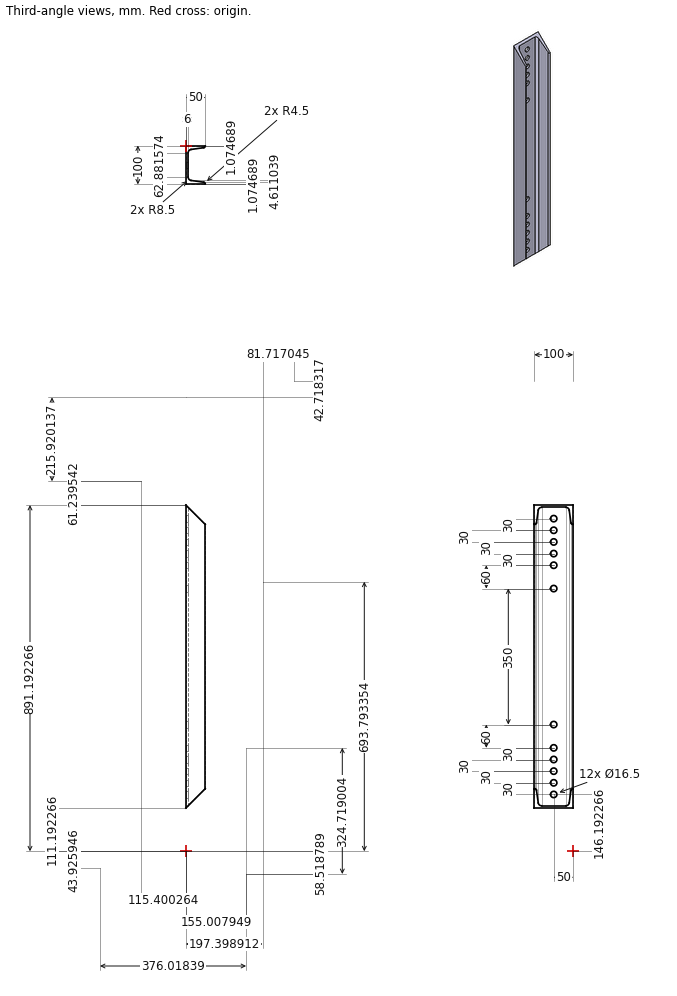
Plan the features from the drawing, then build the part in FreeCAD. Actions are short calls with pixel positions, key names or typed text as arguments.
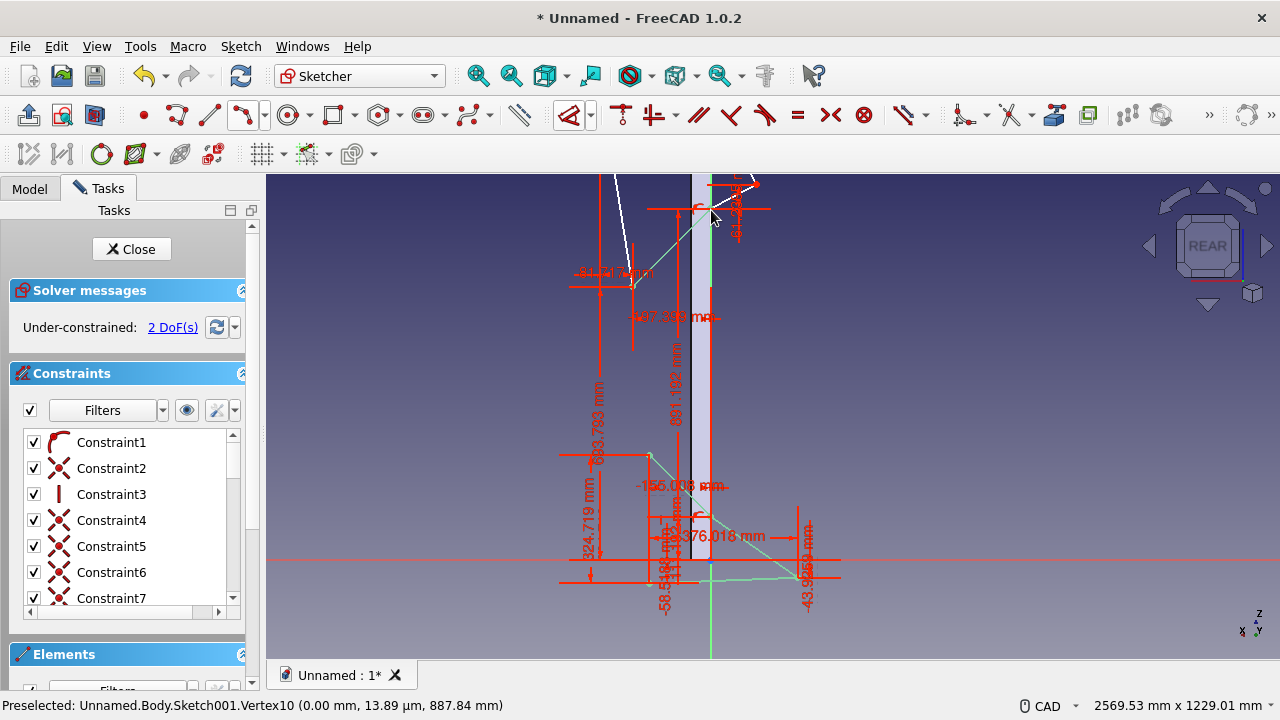
scroll(711, 518, down, 3)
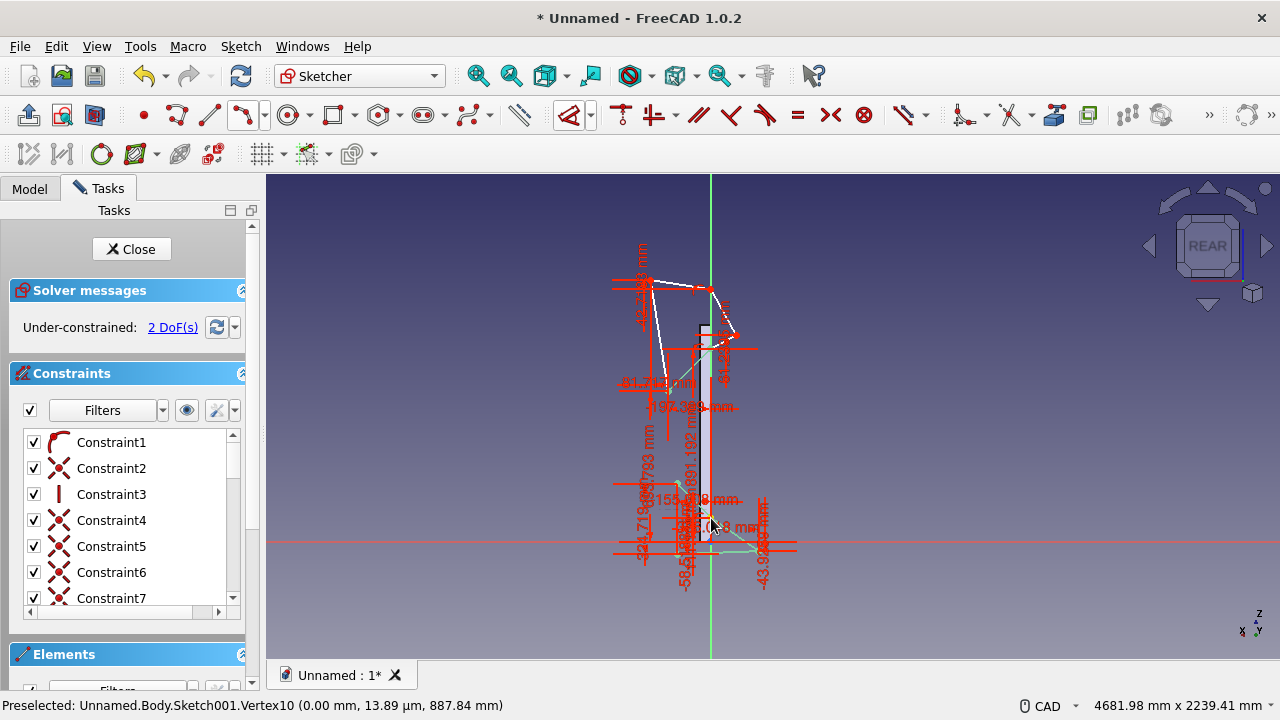
scroll(736, 335, up, 3)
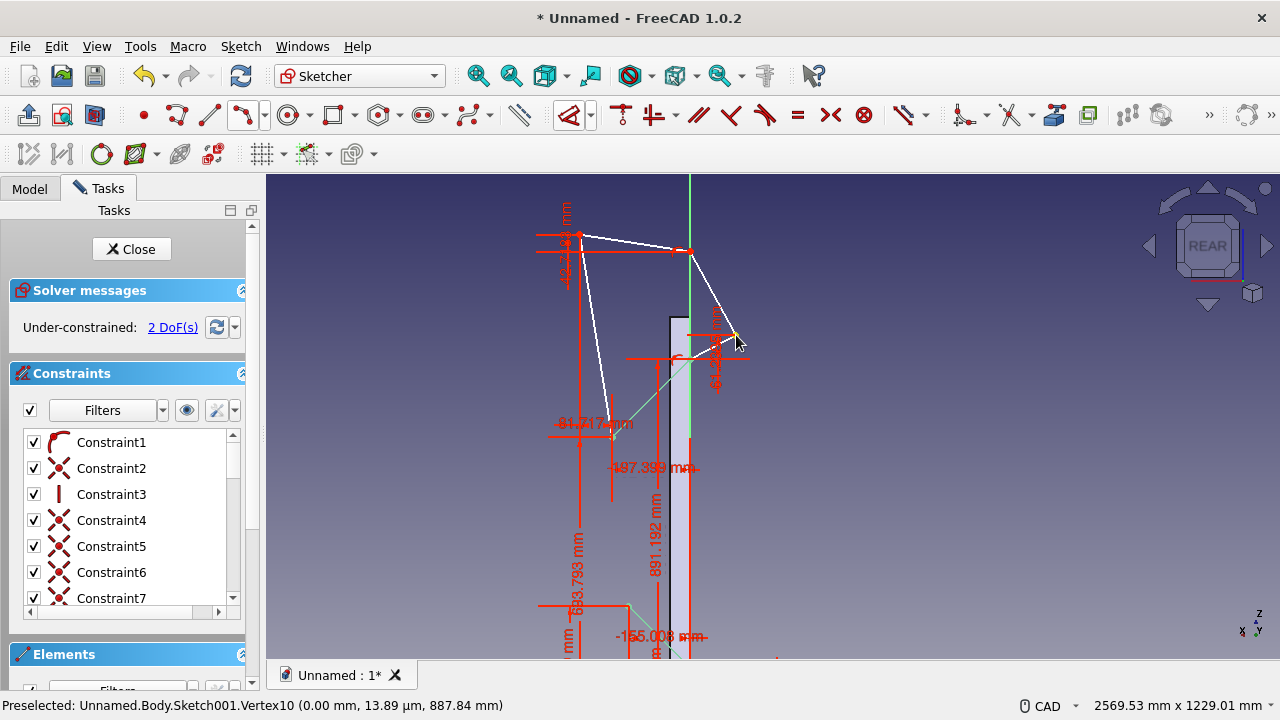
click(736, 335)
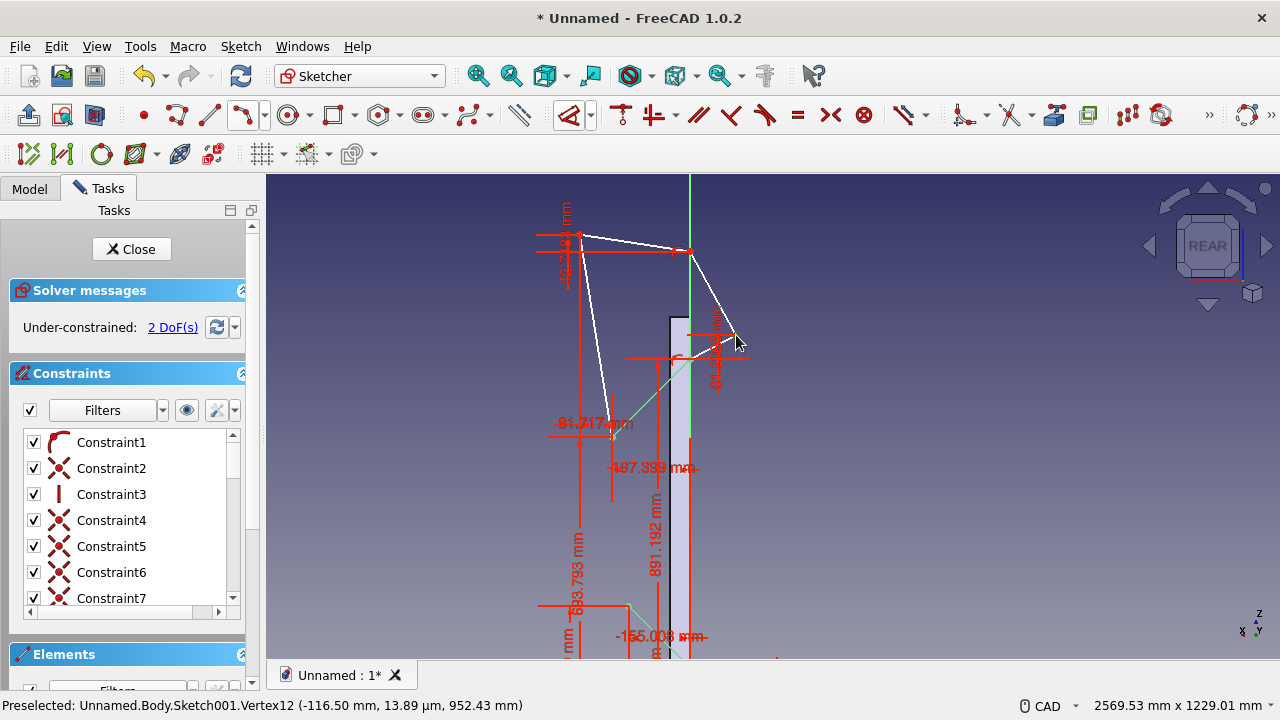
click(590, 116)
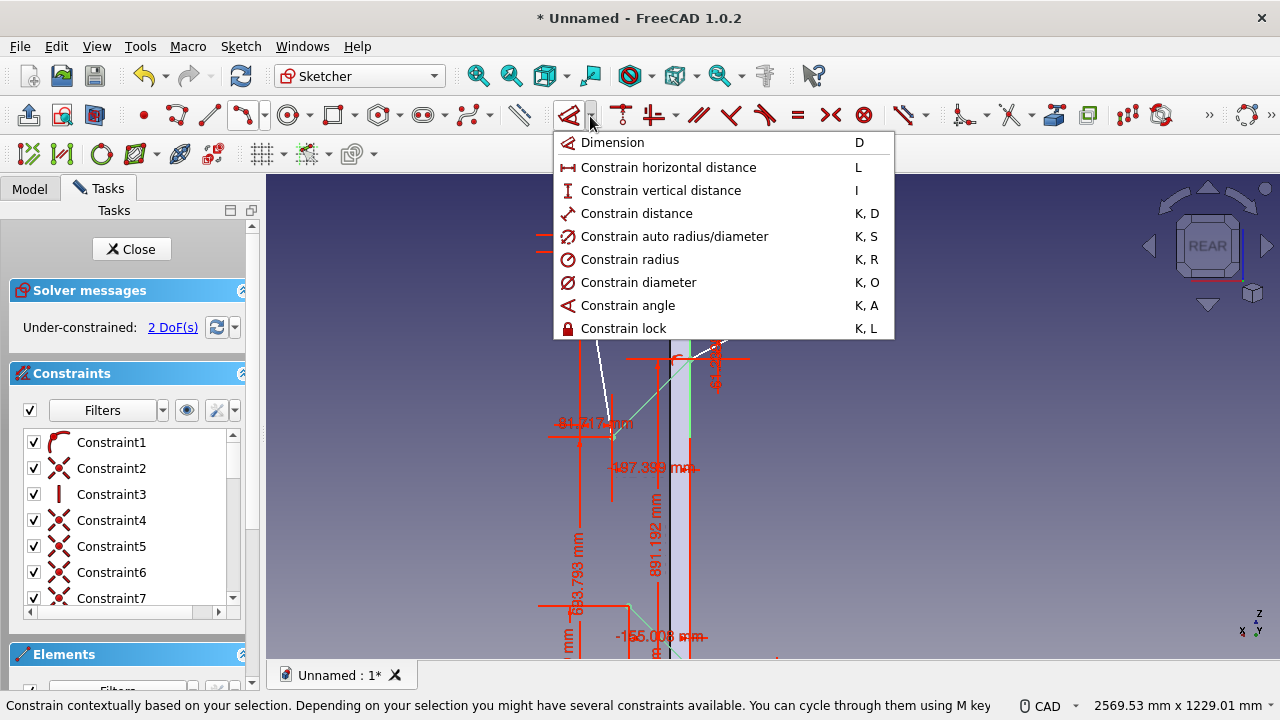
click(724, 168)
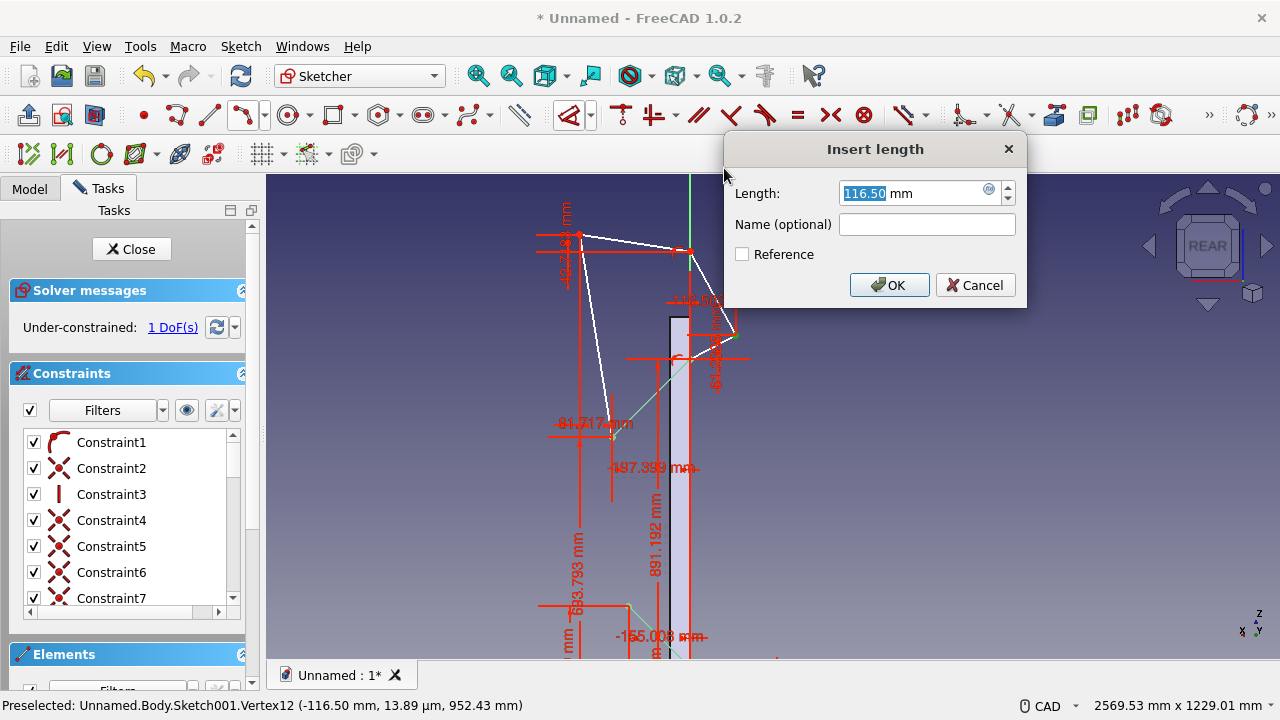
text(115.400264)
key(Return)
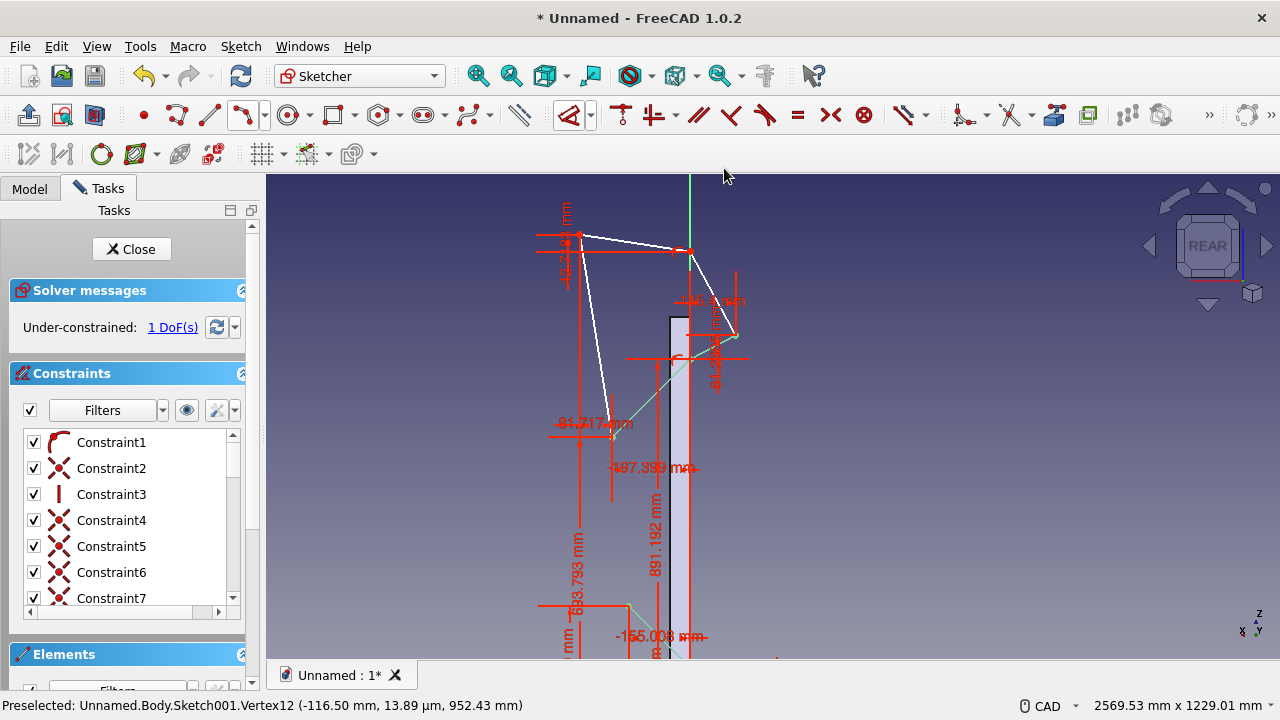
click(704, 277)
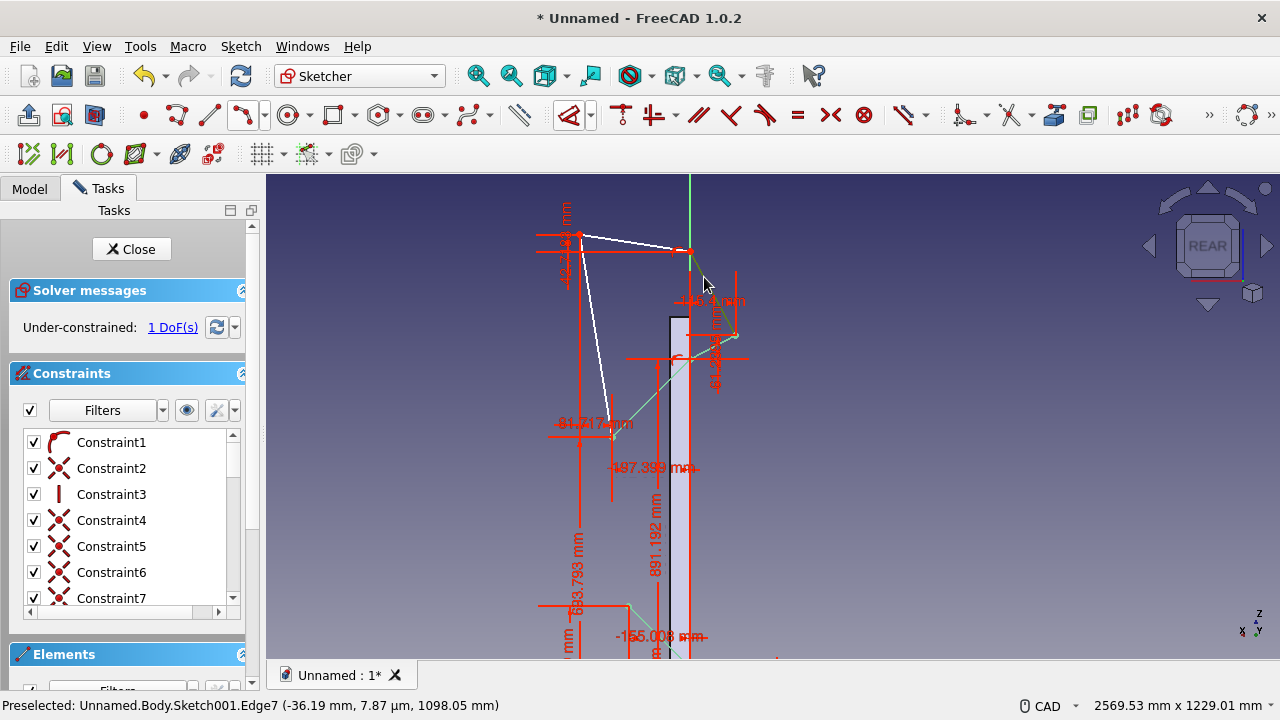
click(590, 116)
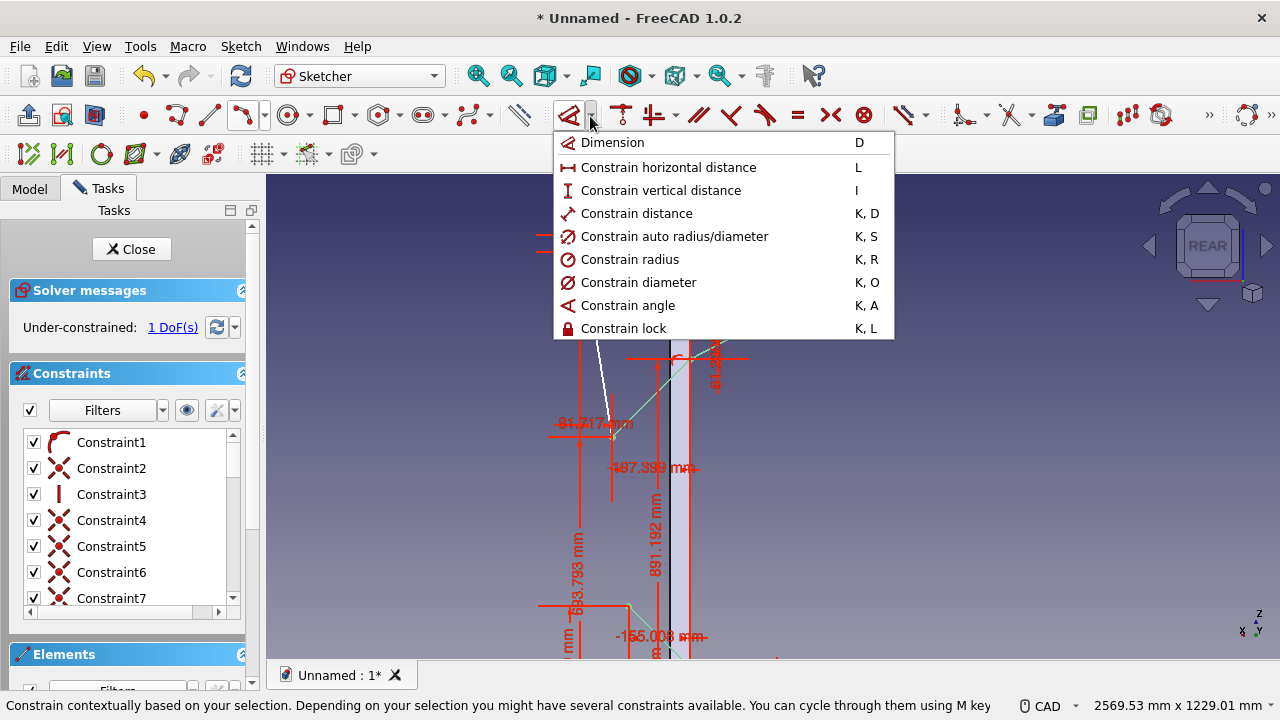
click(724, 190)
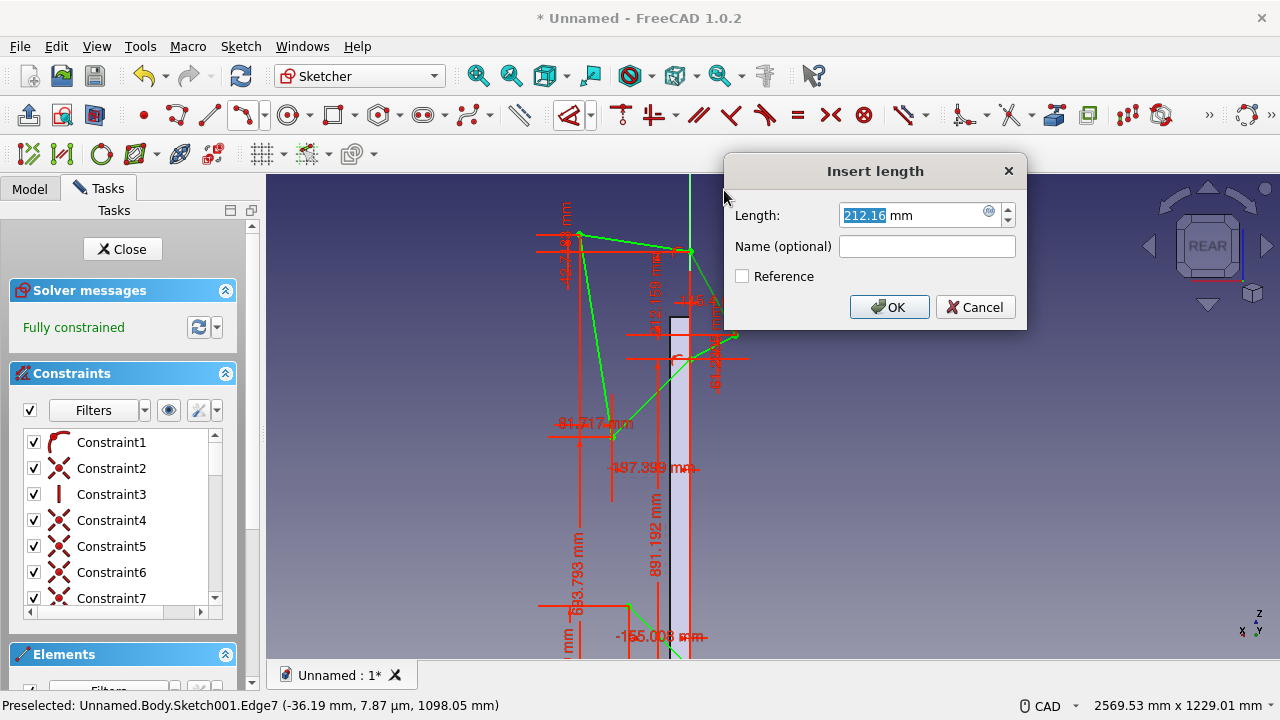
text(215.920137)
key(Return)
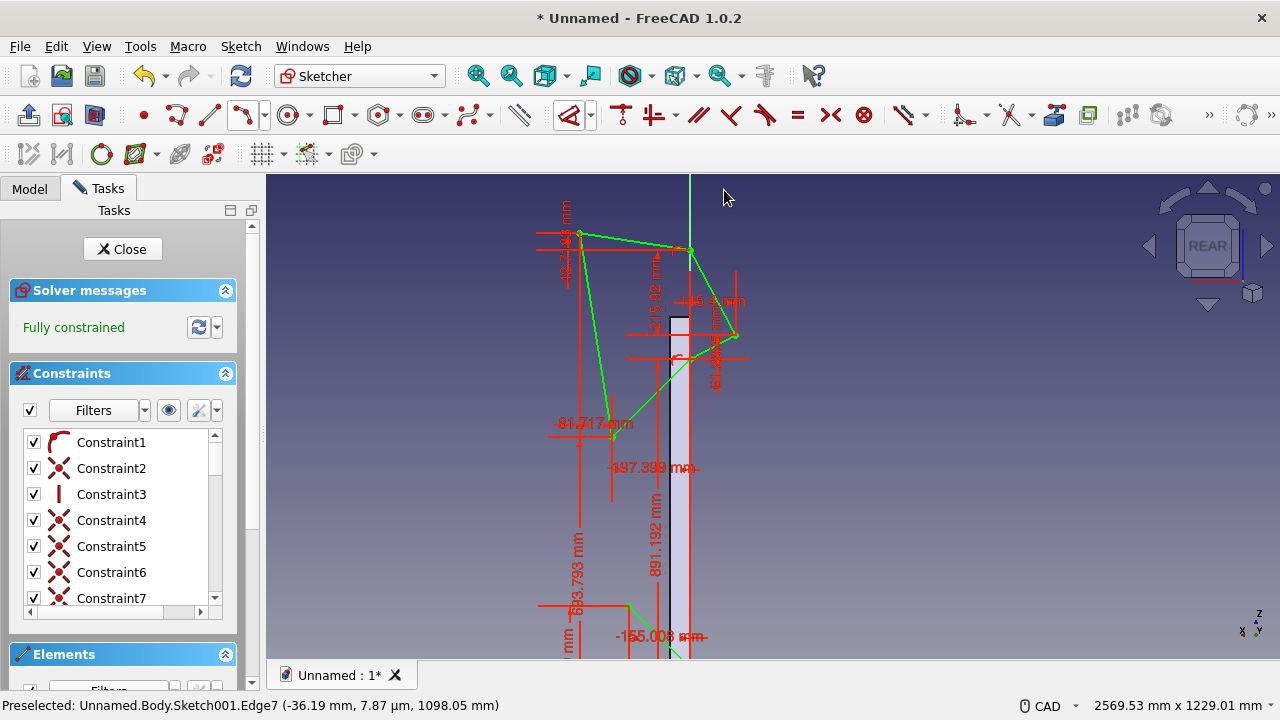
click(123, 249)